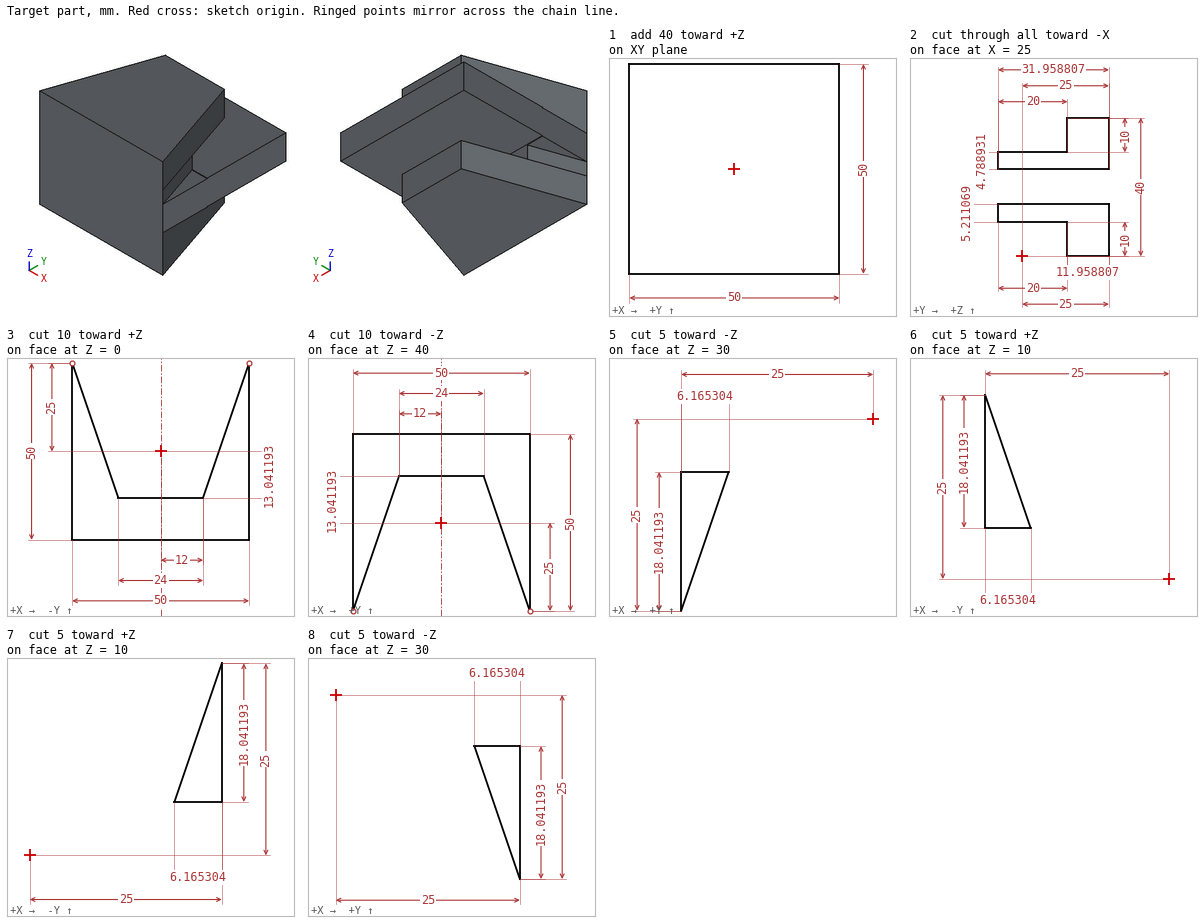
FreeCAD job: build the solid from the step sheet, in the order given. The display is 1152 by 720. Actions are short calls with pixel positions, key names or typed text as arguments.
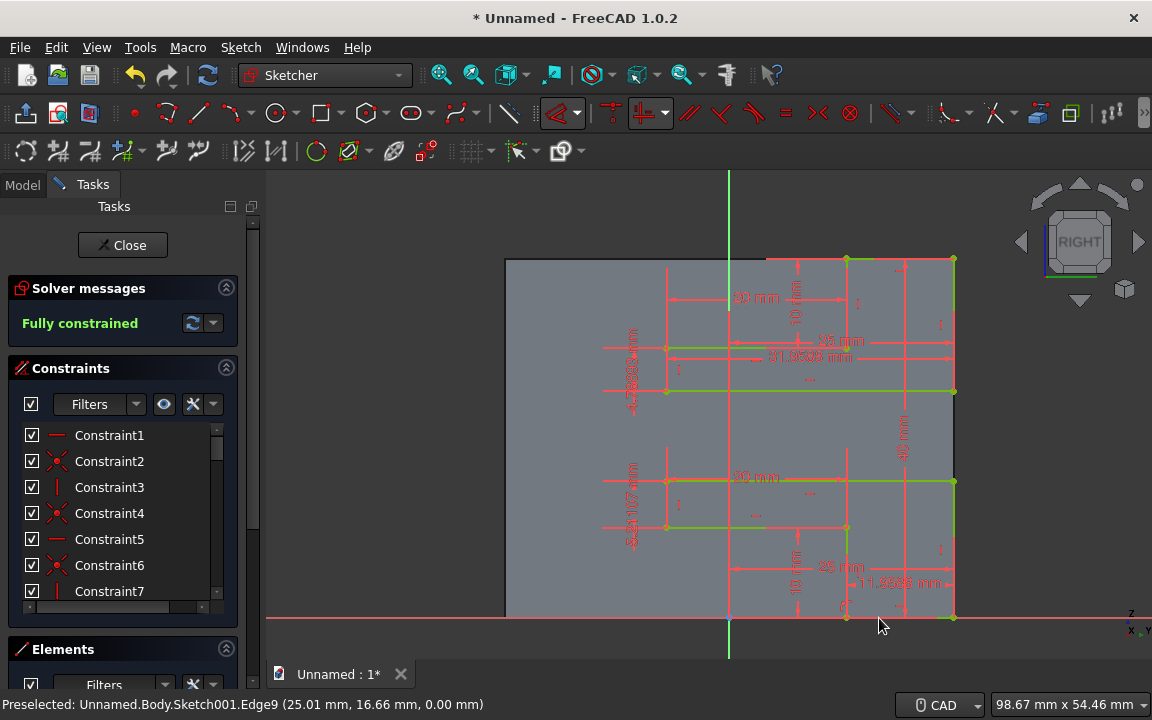
click(123, 245)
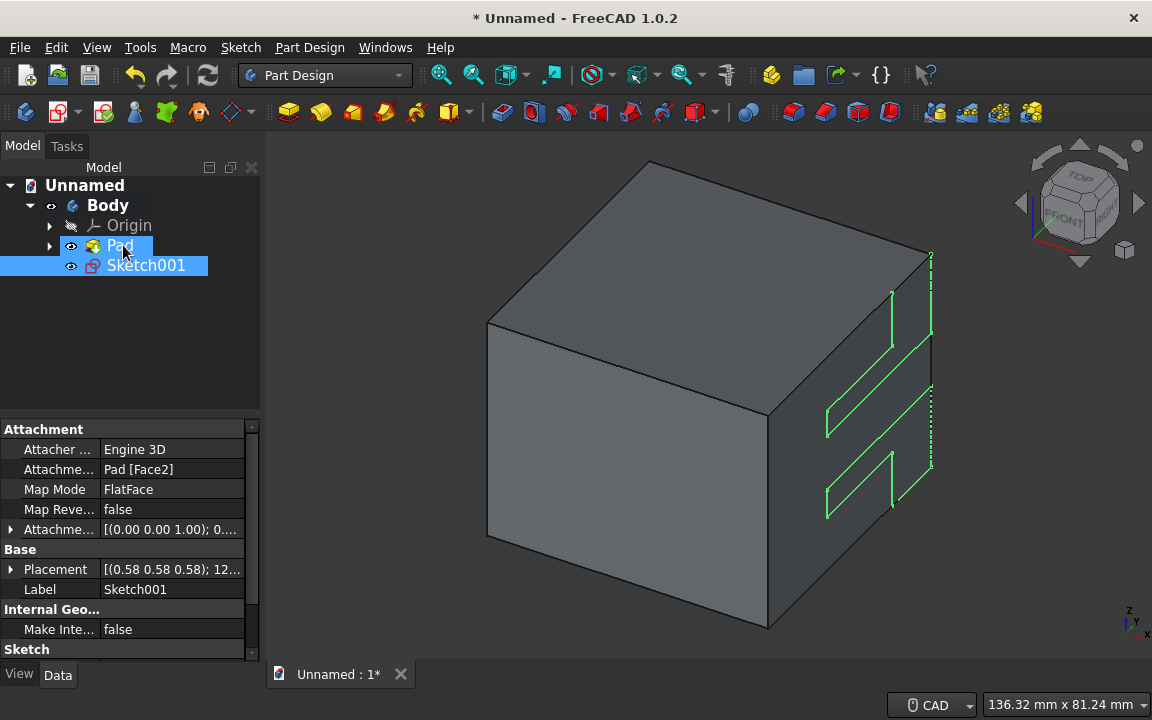
click(504, 112)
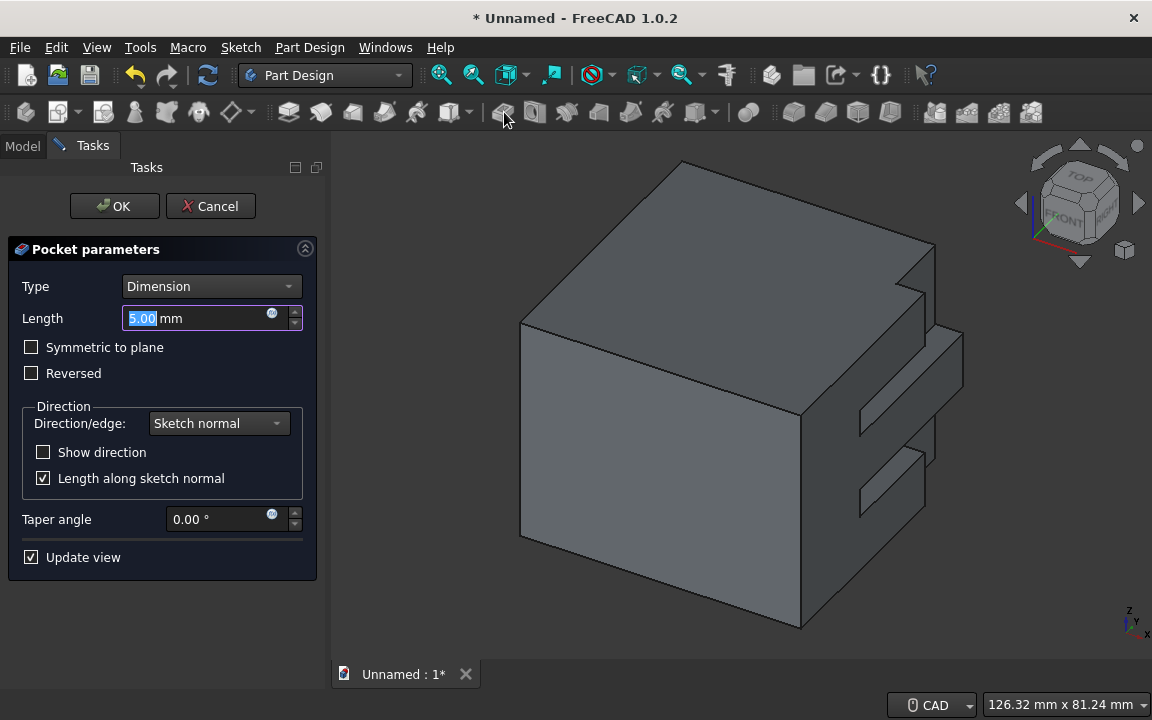
click(212, 286)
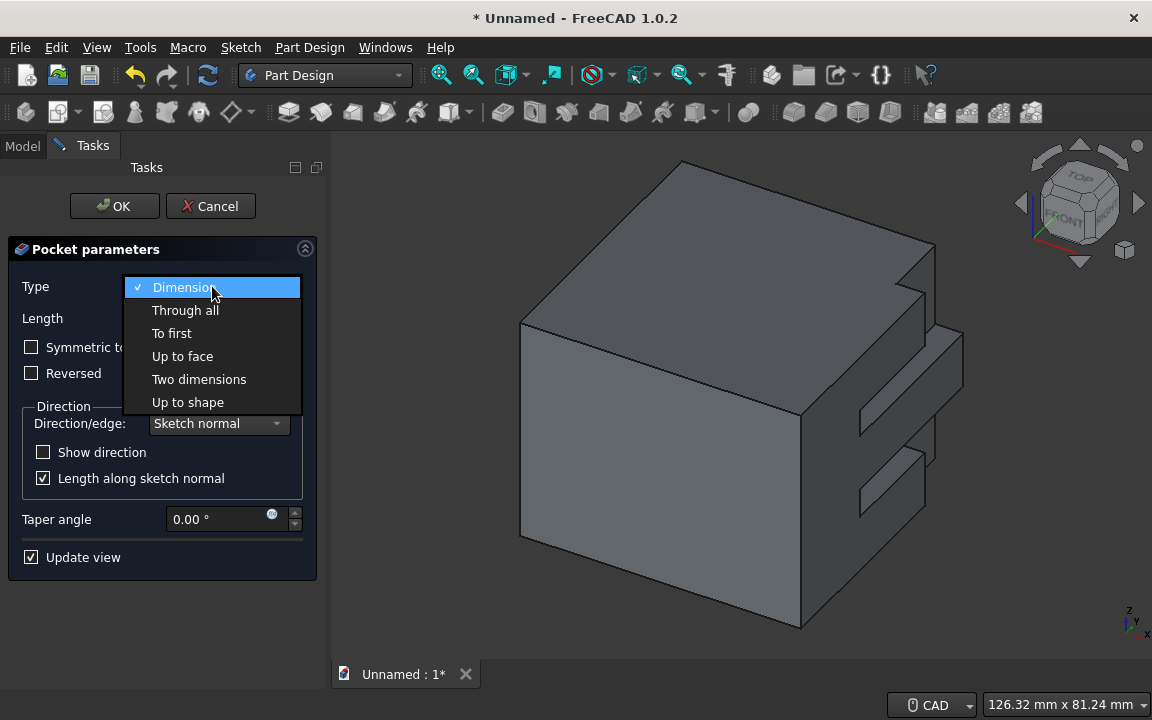
click(212, 310)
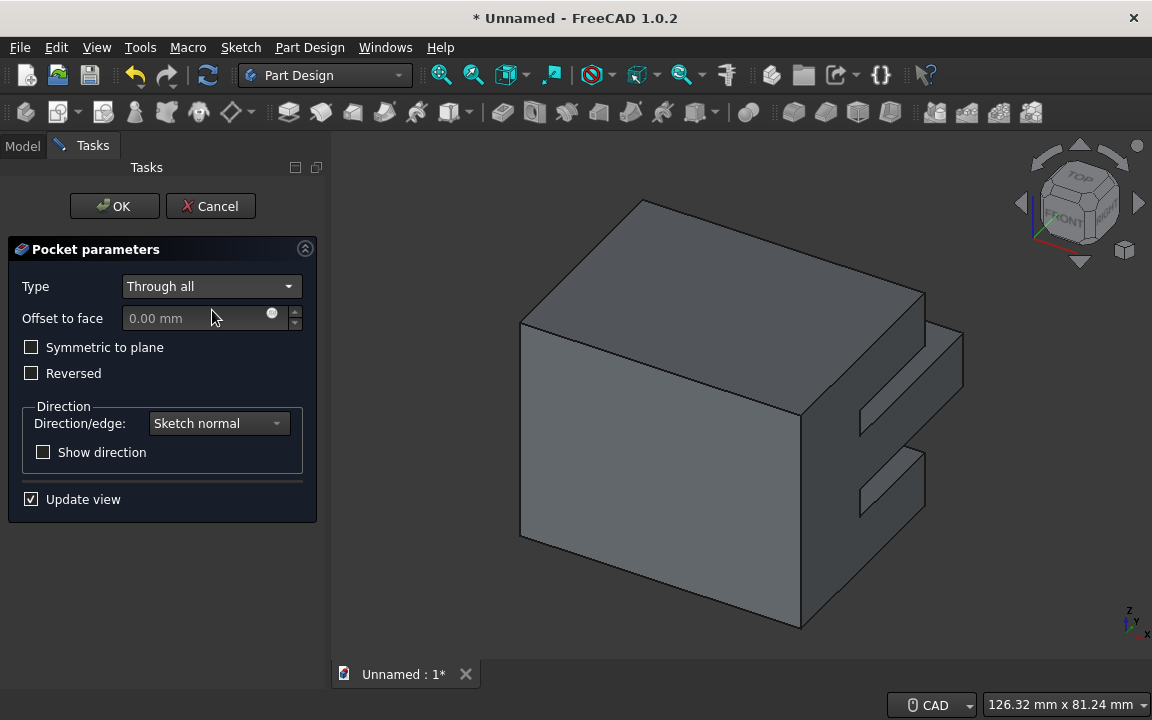
click(115, 206)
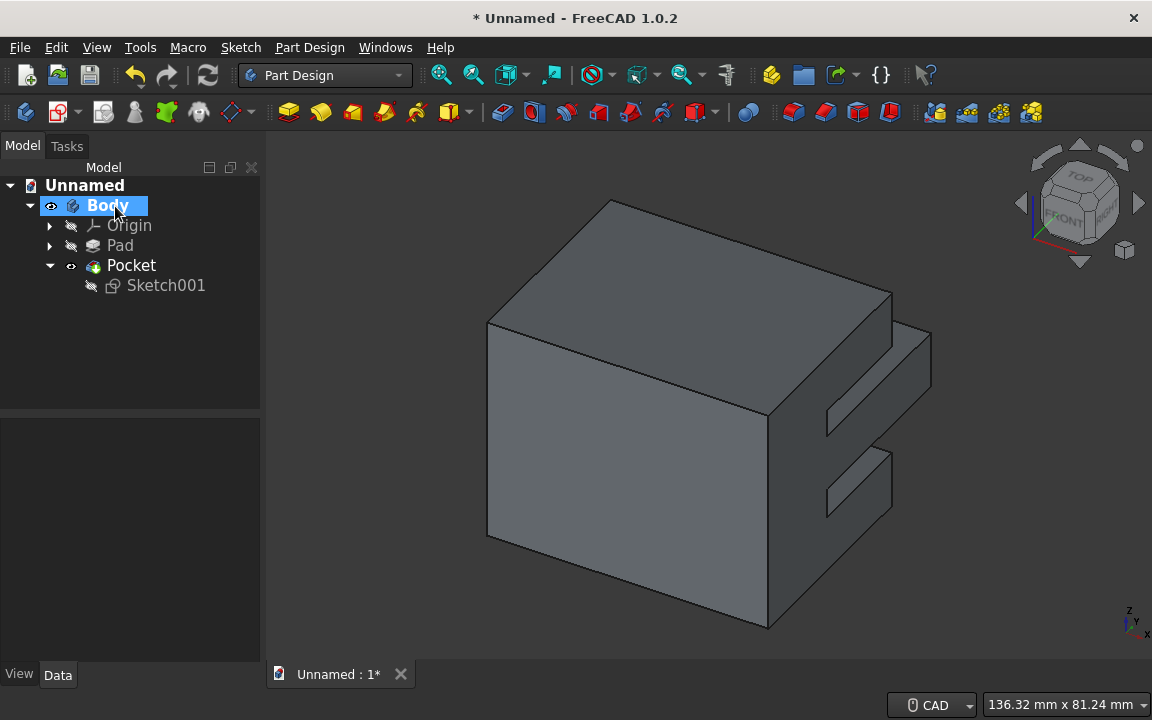
key(5)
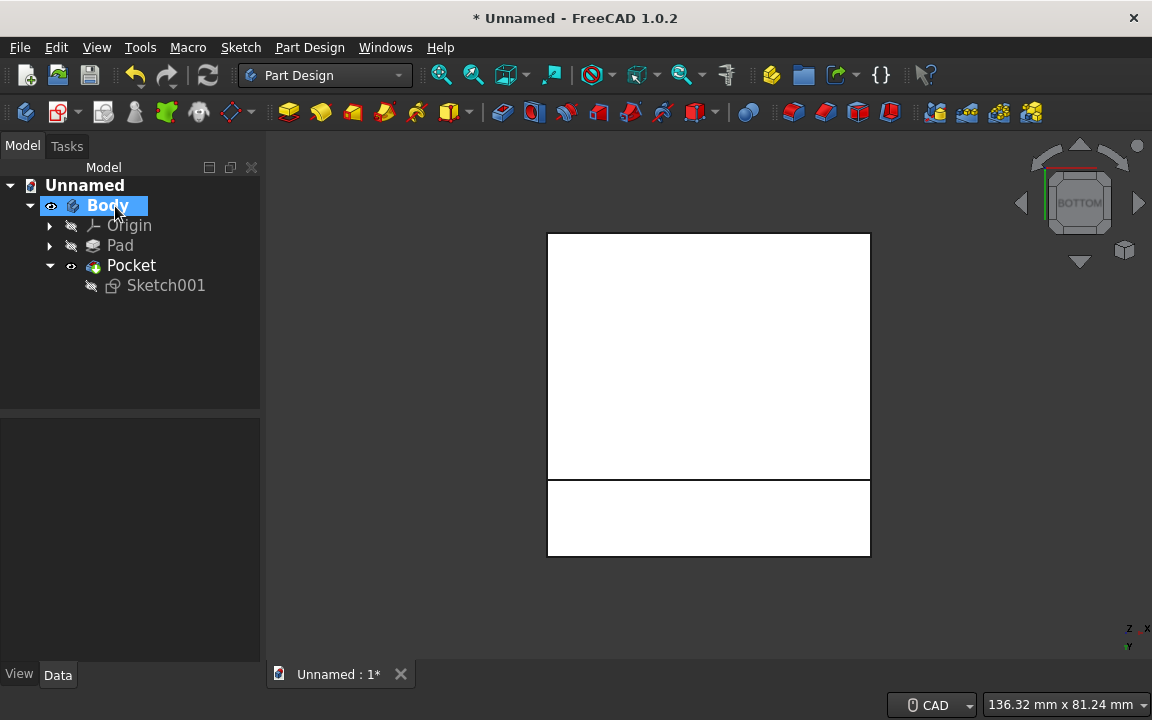
click(709, 355)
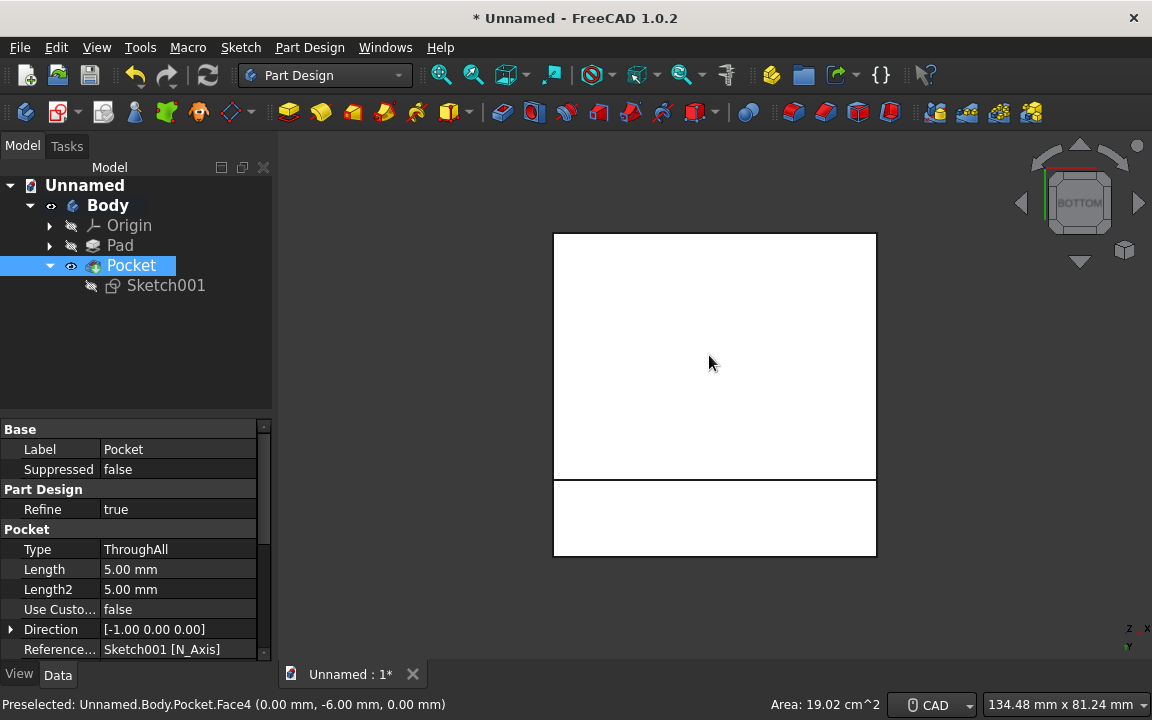
click(58, 112)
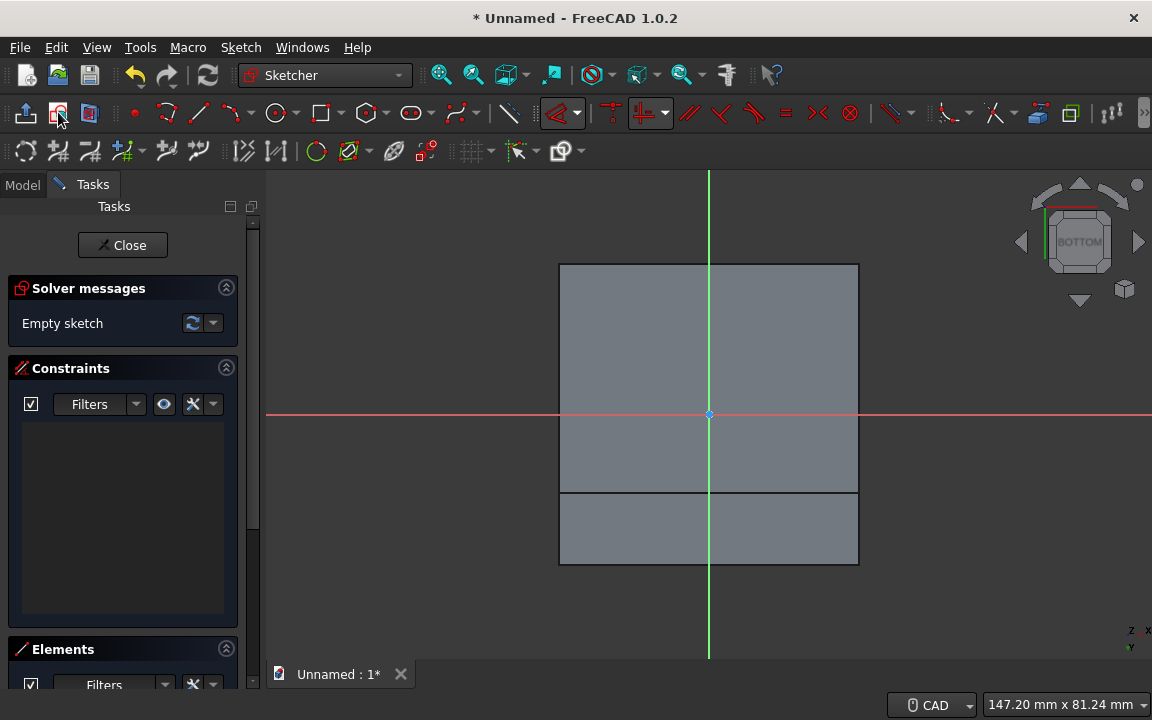
key(g)
key(m)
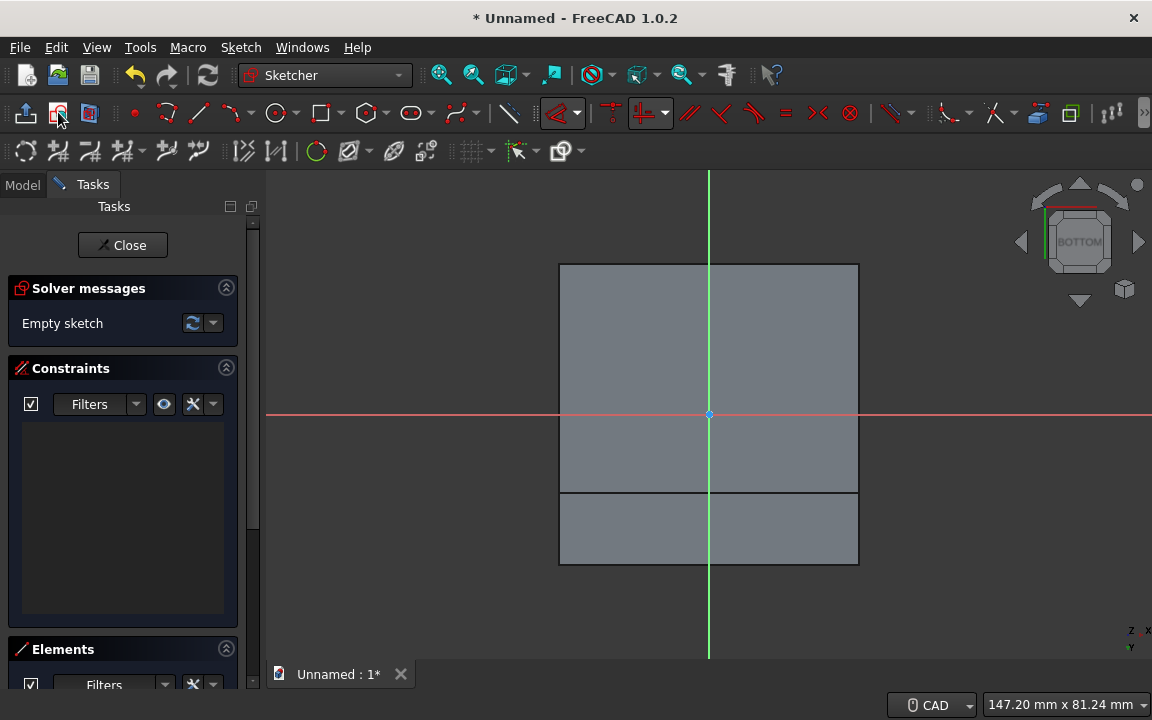
click(781, 493)
click(637, 493)
click(559, 264)
click(559, 565)
click(859, 565)
click(859, 264)
click(781, 494)
key(Escape)
key(Escape)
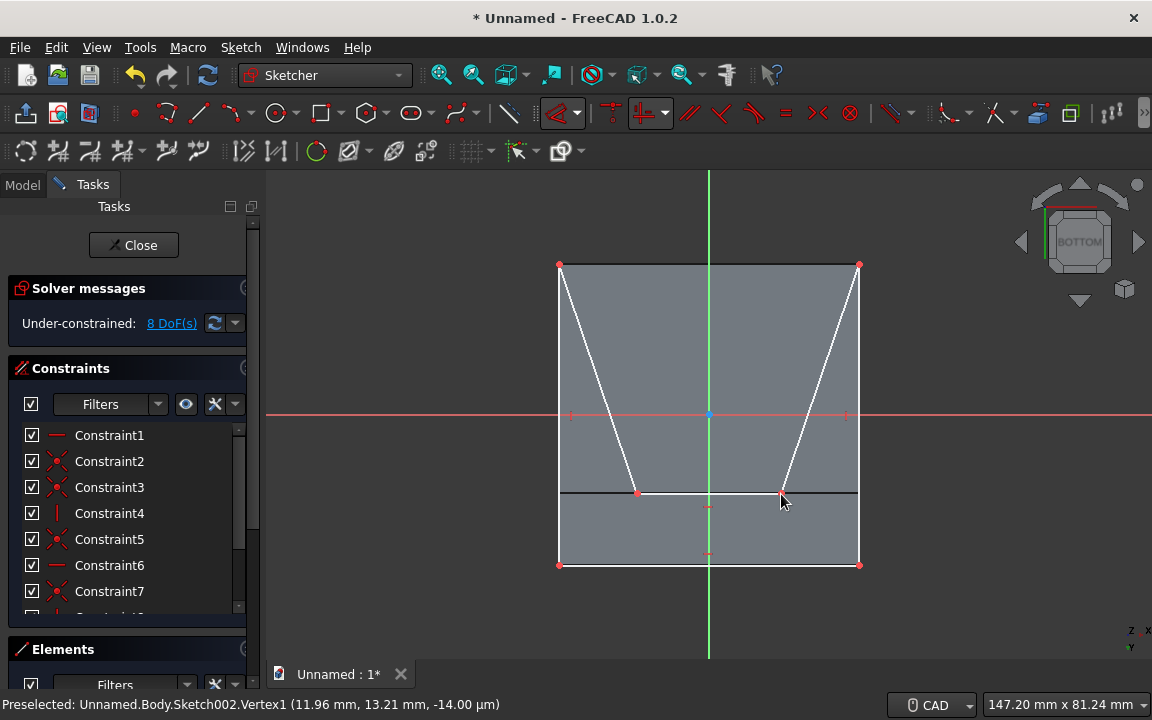
click(559, 265)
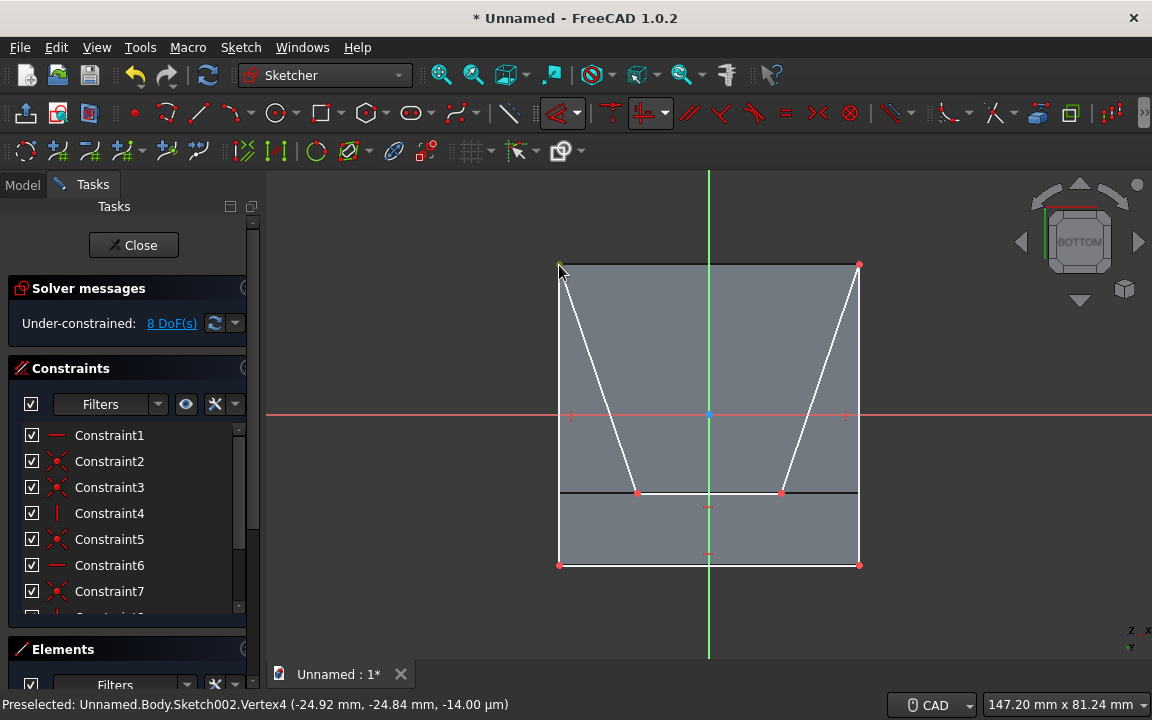
click(859, 265)